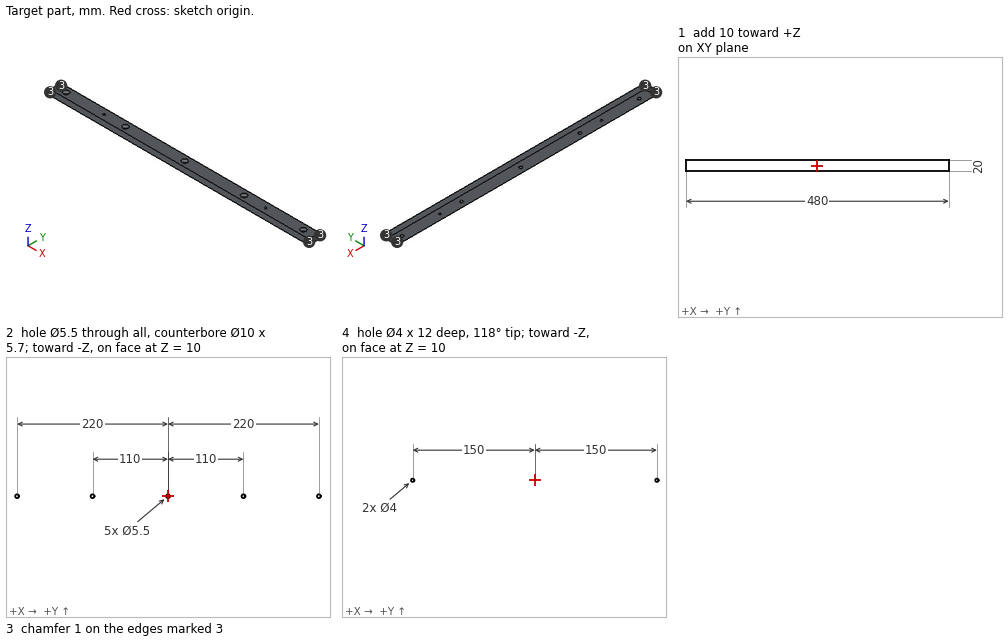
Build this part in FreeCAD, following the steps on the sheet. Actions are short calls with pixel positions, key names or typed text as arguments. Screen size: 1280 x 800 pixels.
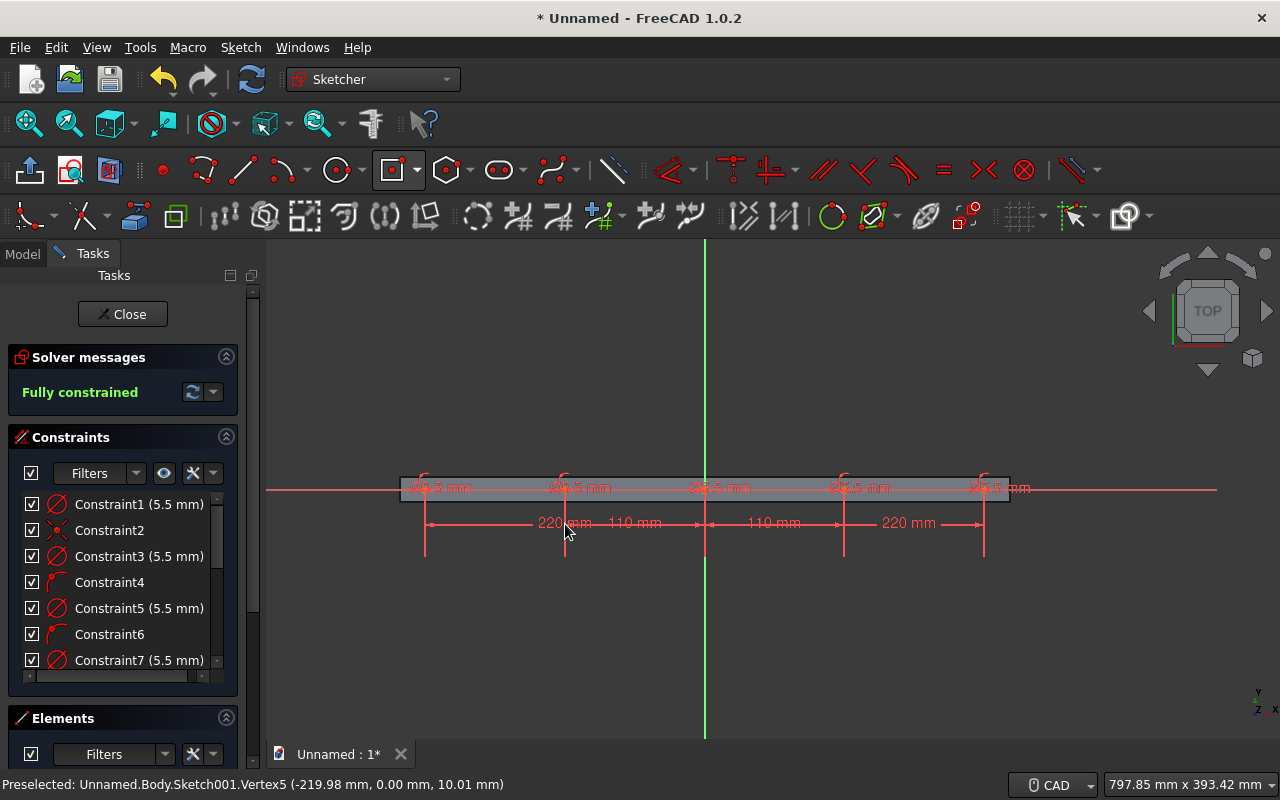
click(123, 314)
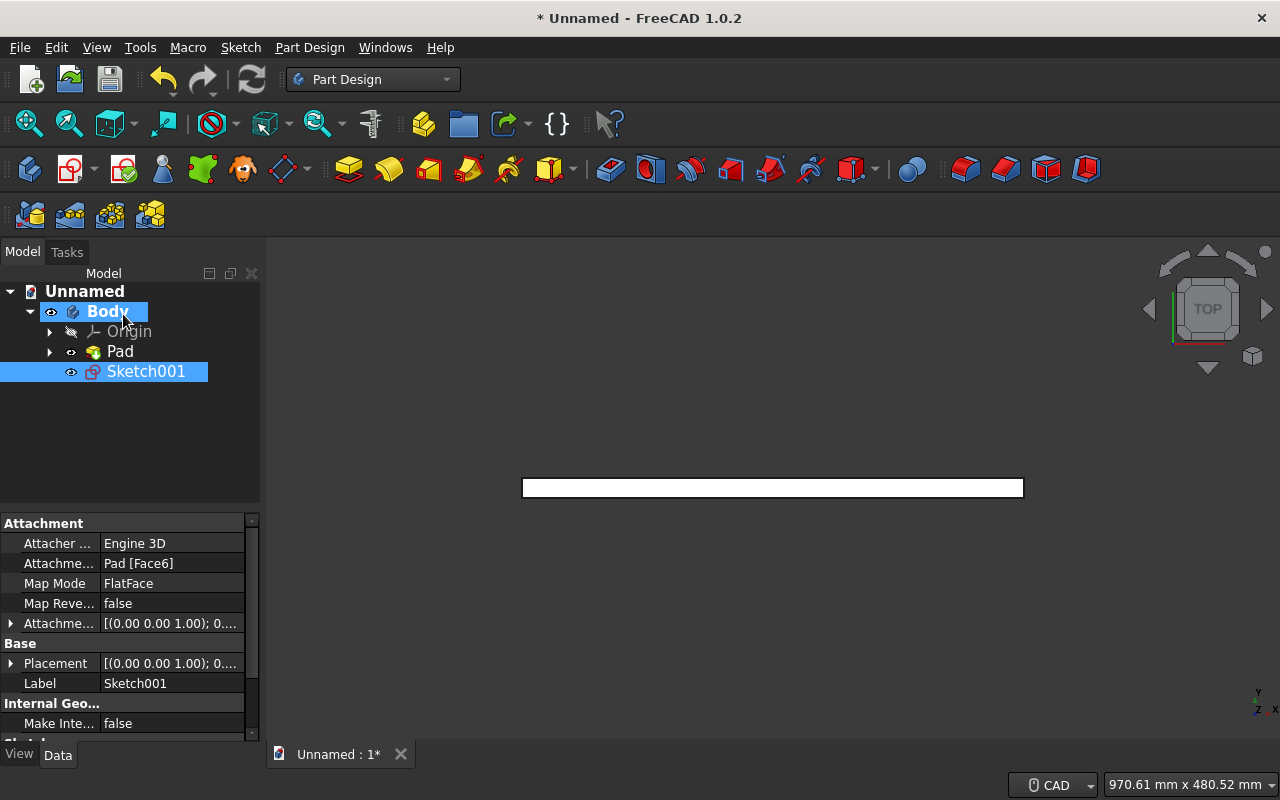
click(652, 170)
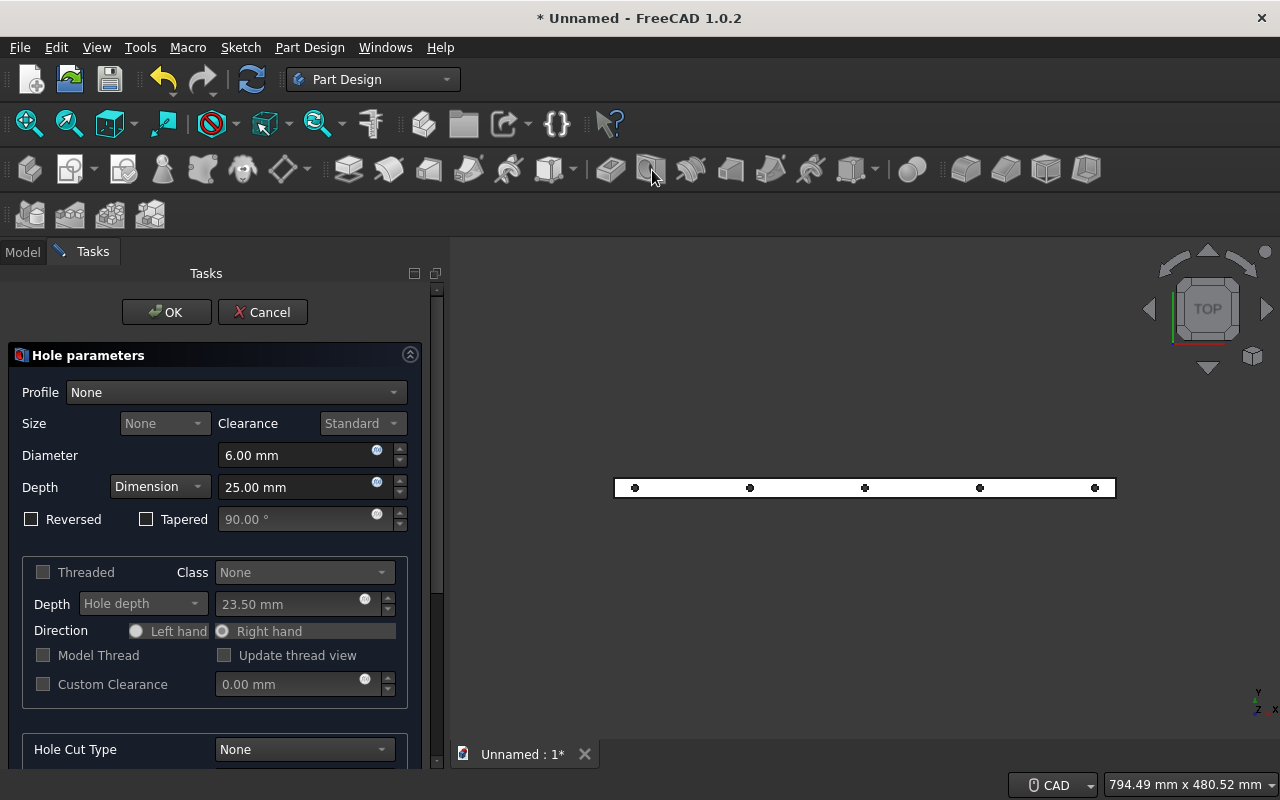
triple_click(305, 455)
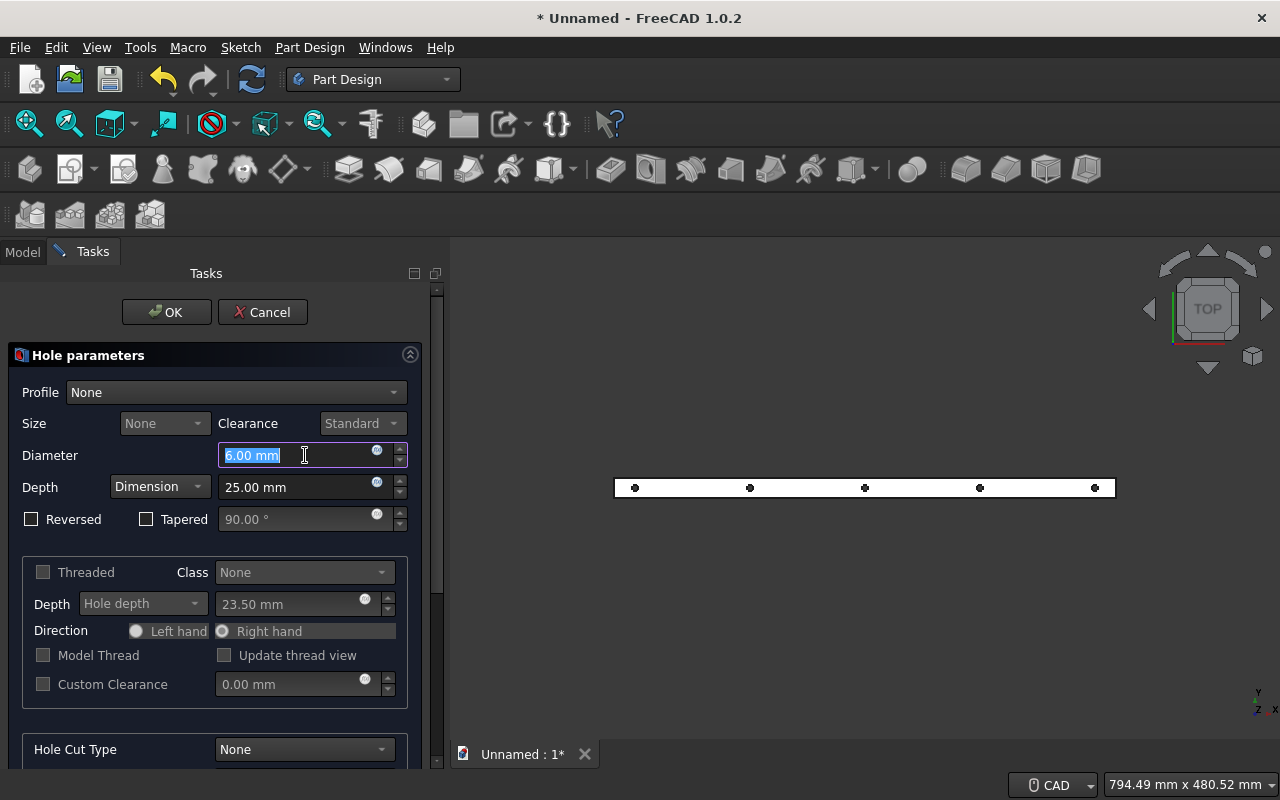
text(5.5)
key(Tab)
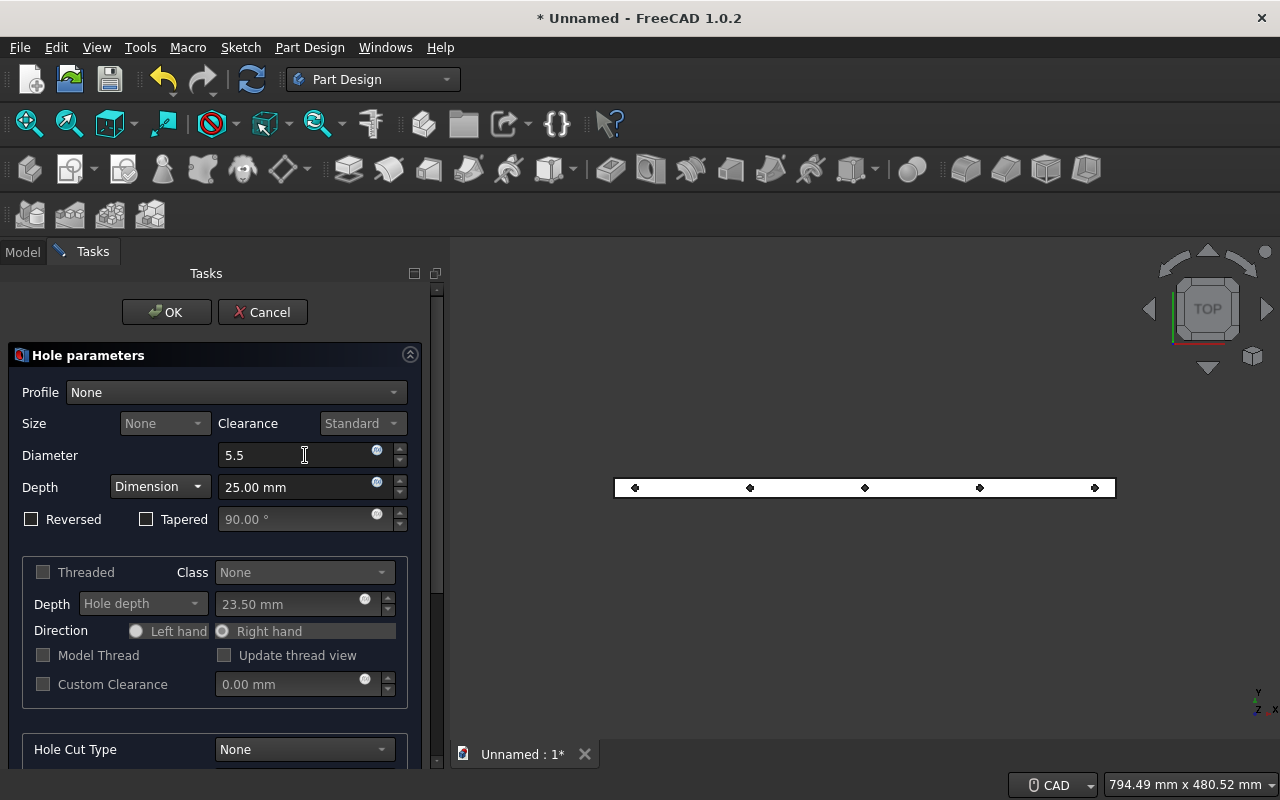
click(161, 486)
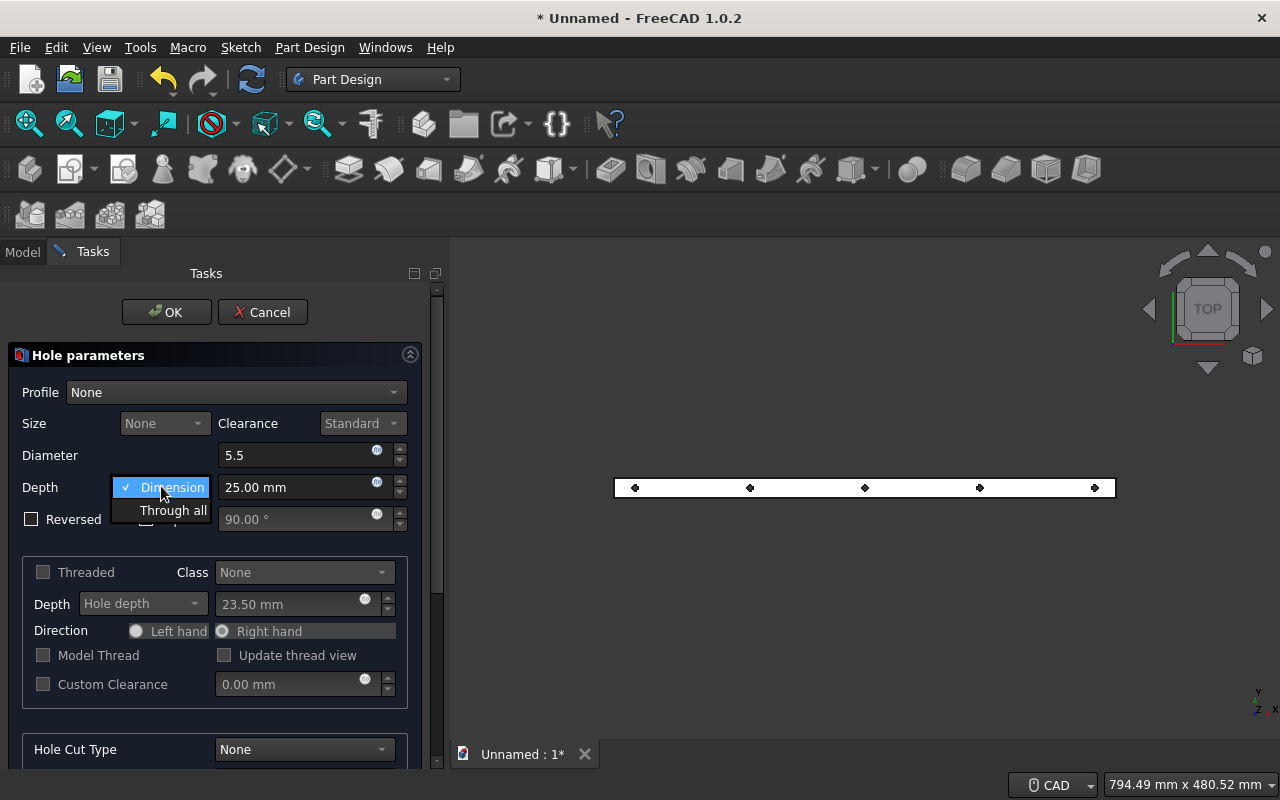
click(160, 510)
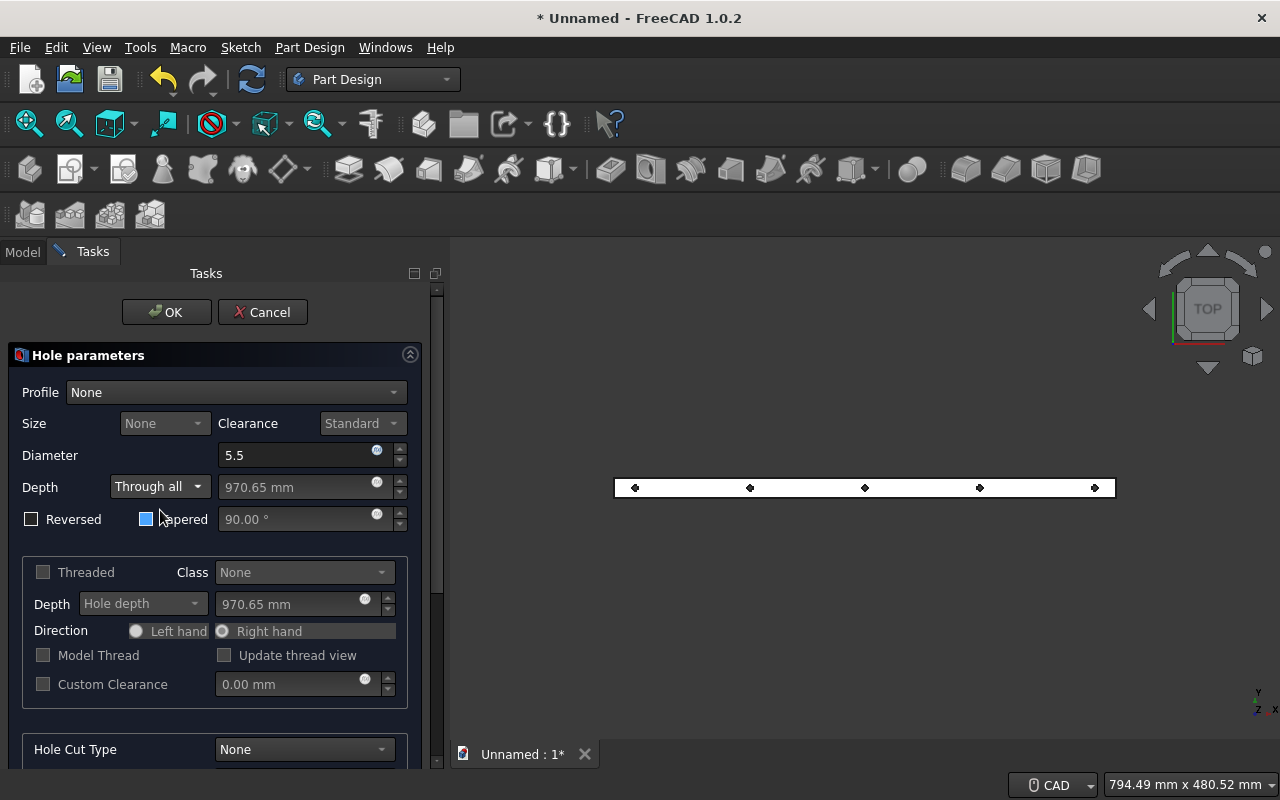
click(306, 750)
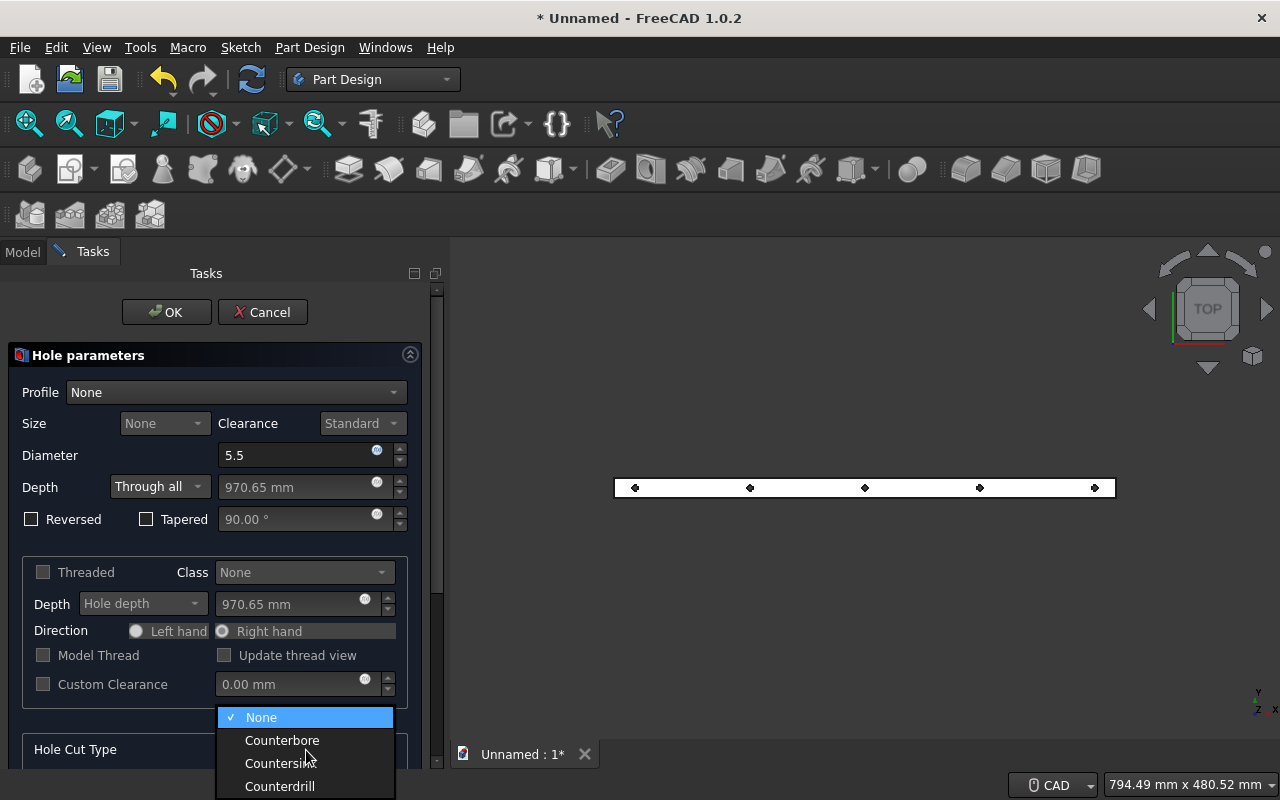
click(304, 740)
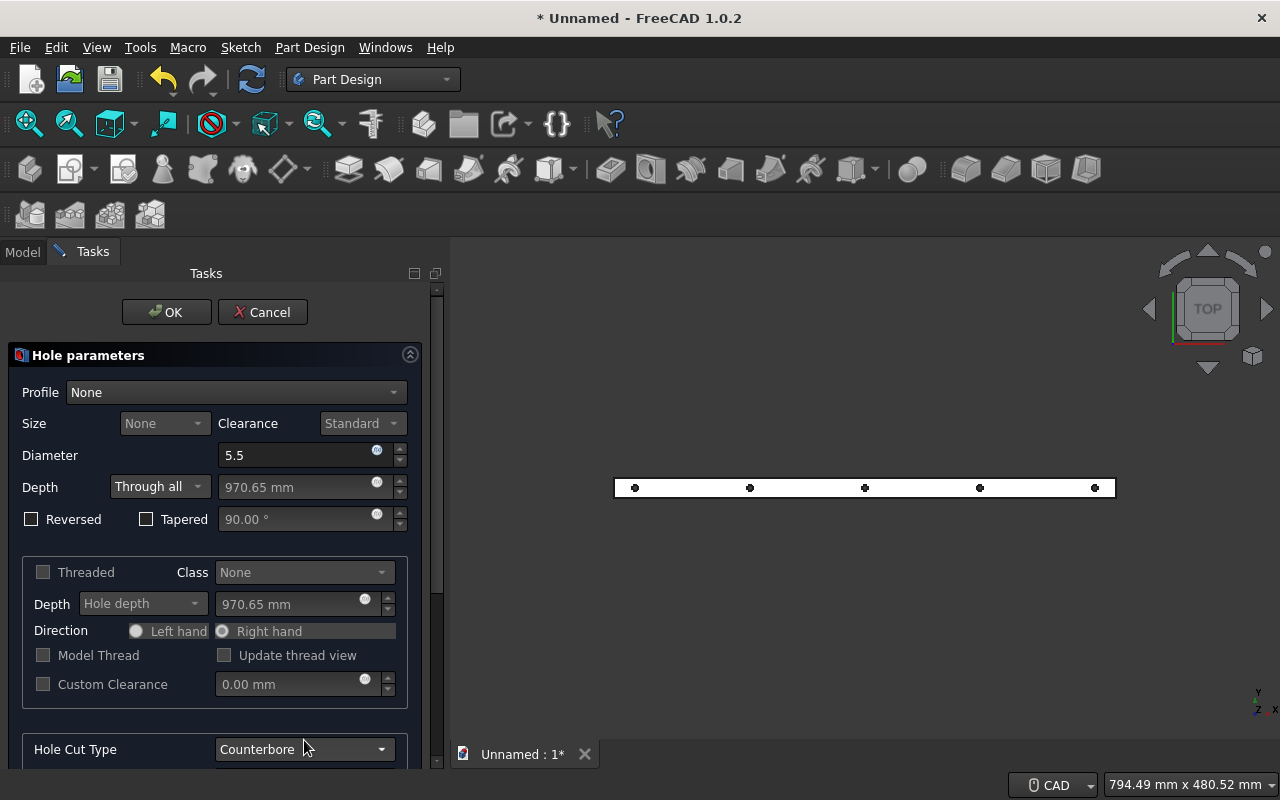
scroll(437, 526, down, 2)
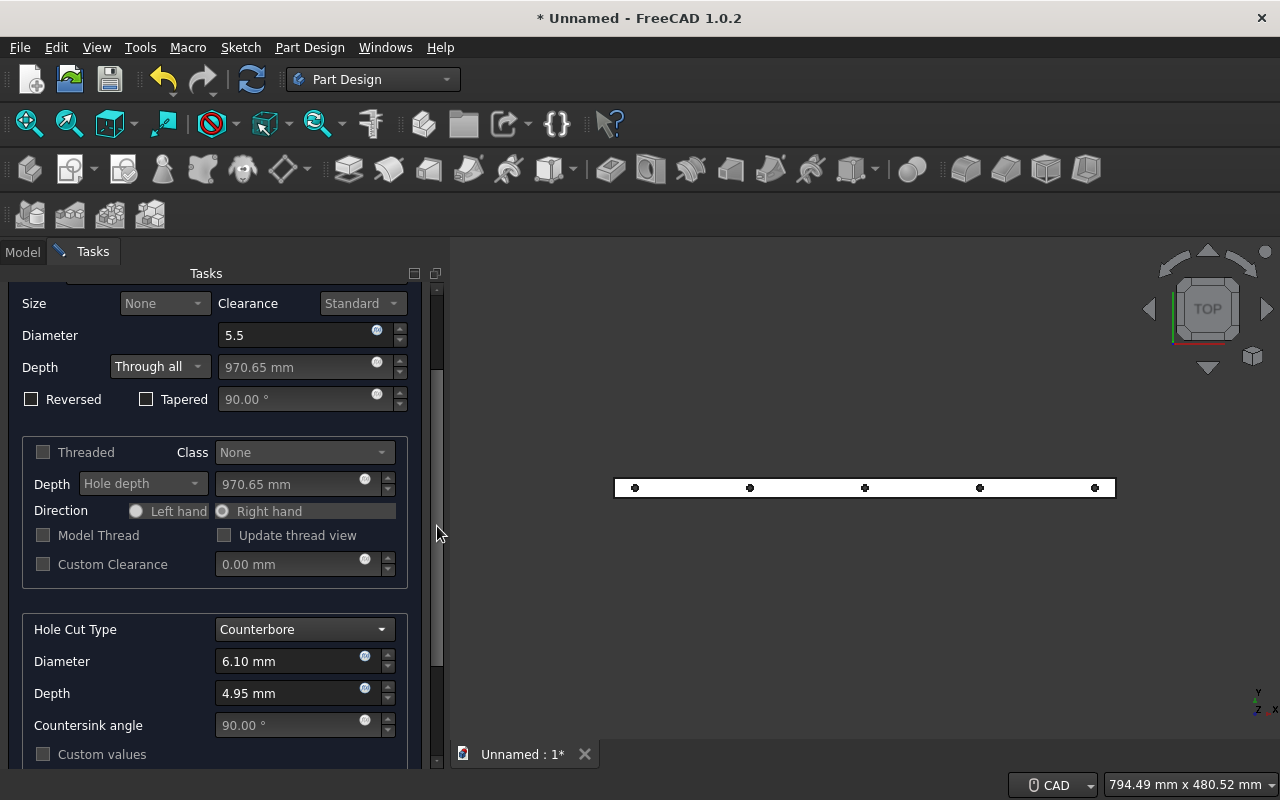
triple_click(298, 661)